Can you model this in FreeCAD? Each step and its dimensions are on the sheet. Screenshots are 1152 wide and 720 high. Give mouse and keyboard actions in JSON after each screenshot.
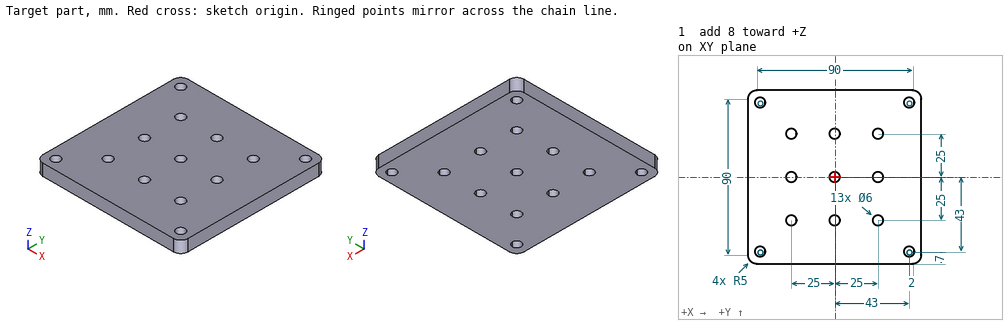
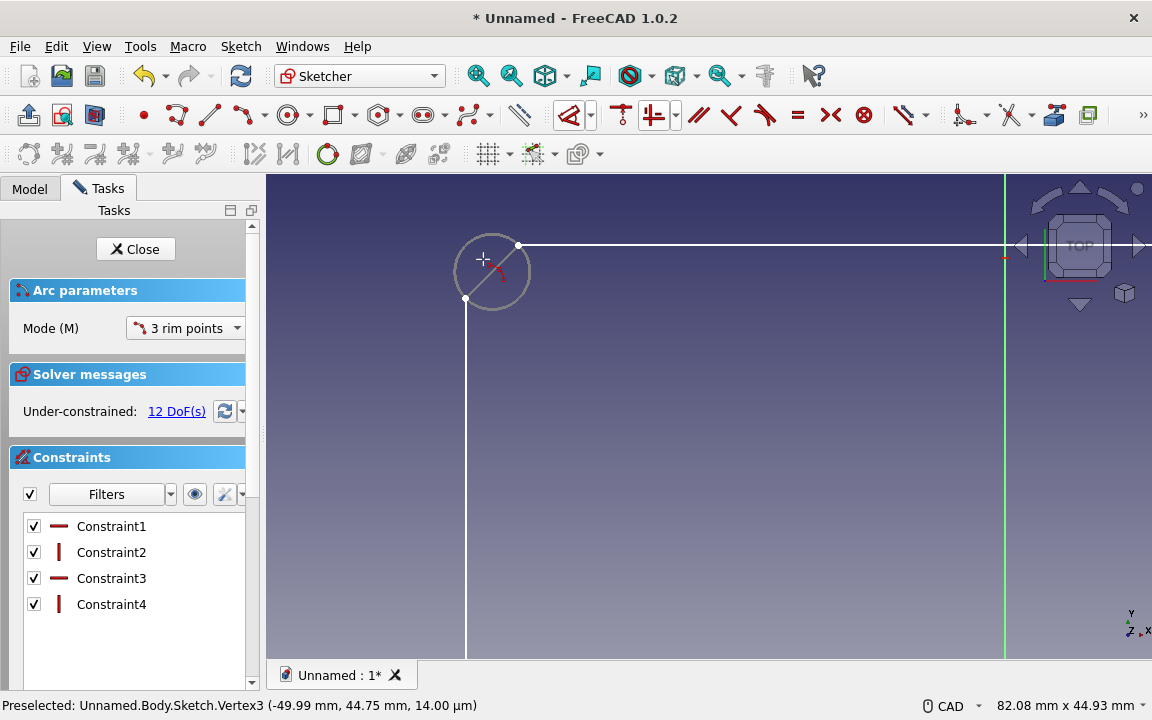
{"action": "left_click", "coordinate": [481, 257]}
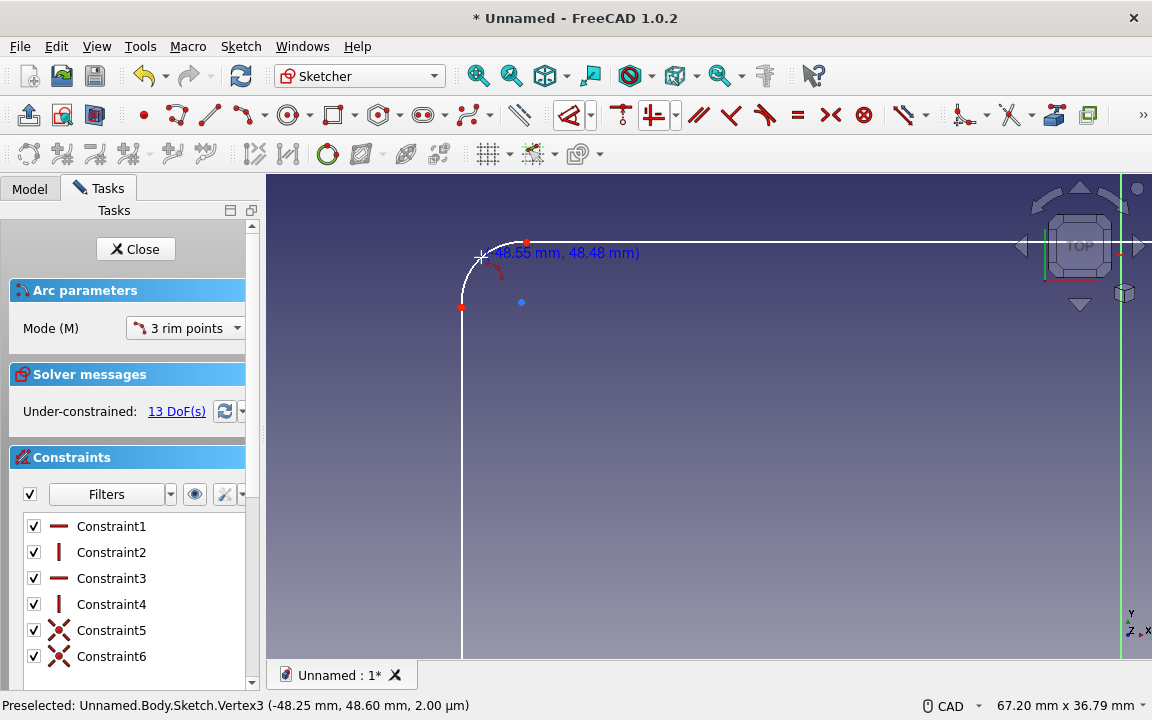
{"action": "scroll", "coordinate": [483, 259], "scroll_direction": "down", "scroll_amount": 7}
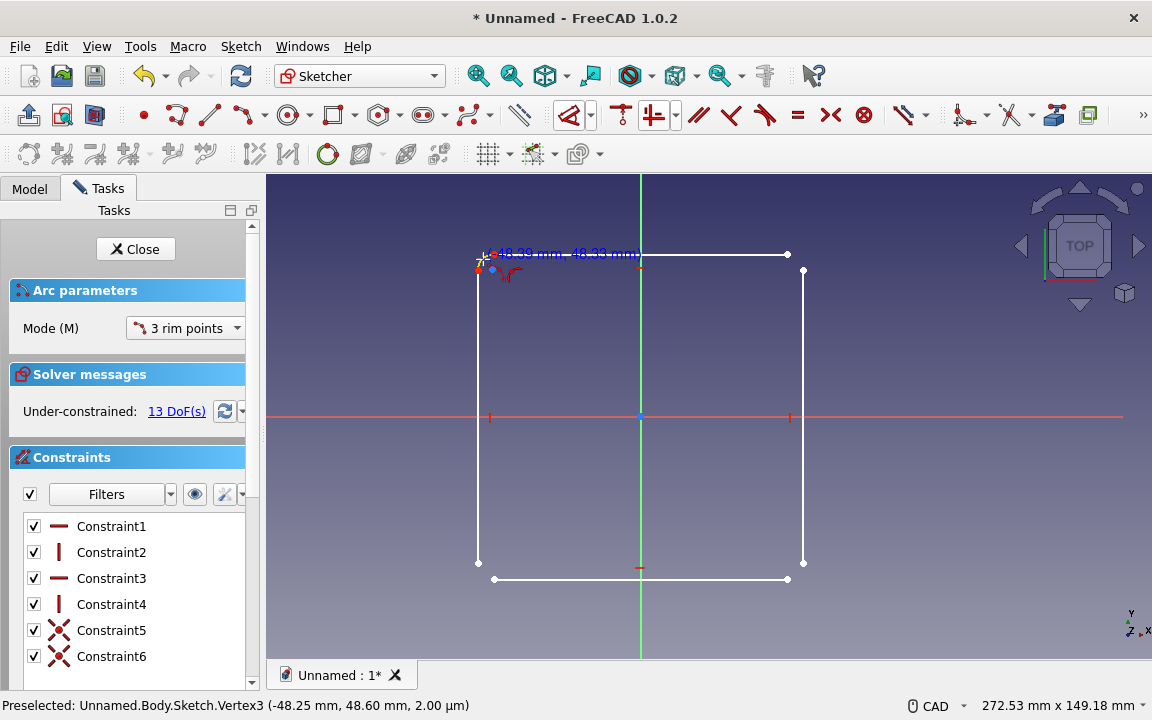
{"action": "left_click", "coordinate": [478, 564]}
{"action": "left_click", "coordinate": [494, 580]}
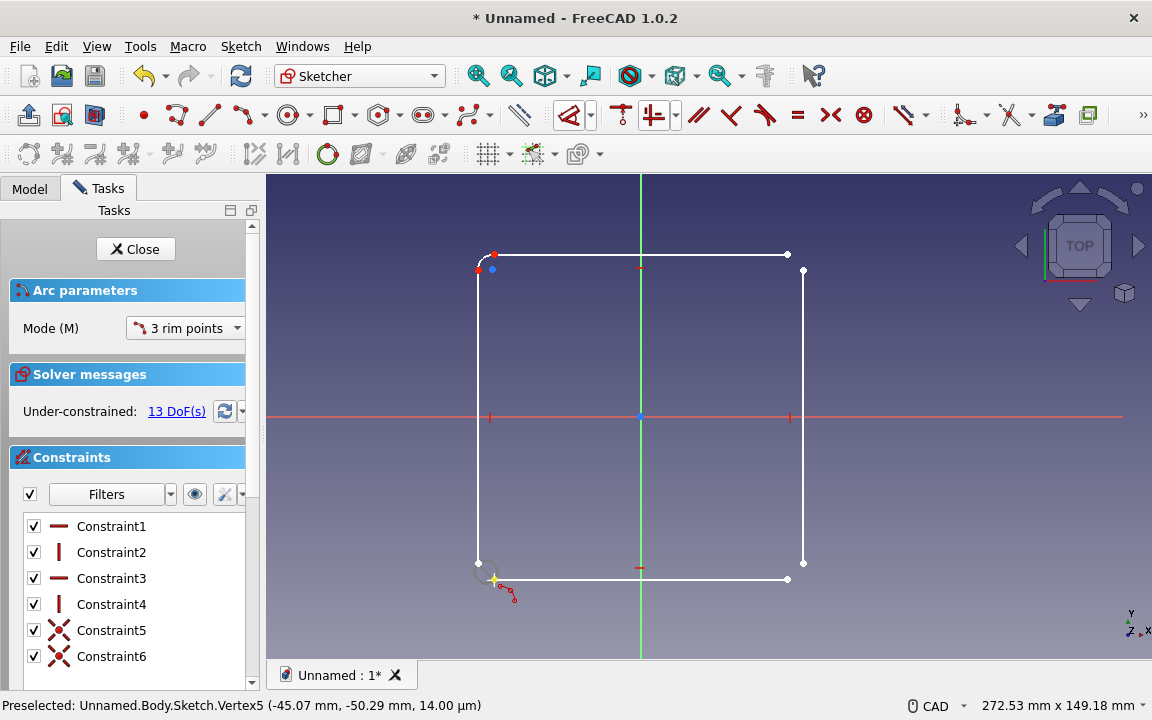
{"action": "scroll", "coordinate": [483, 574], "scroll_direction": "up", "scroll_amount": 7}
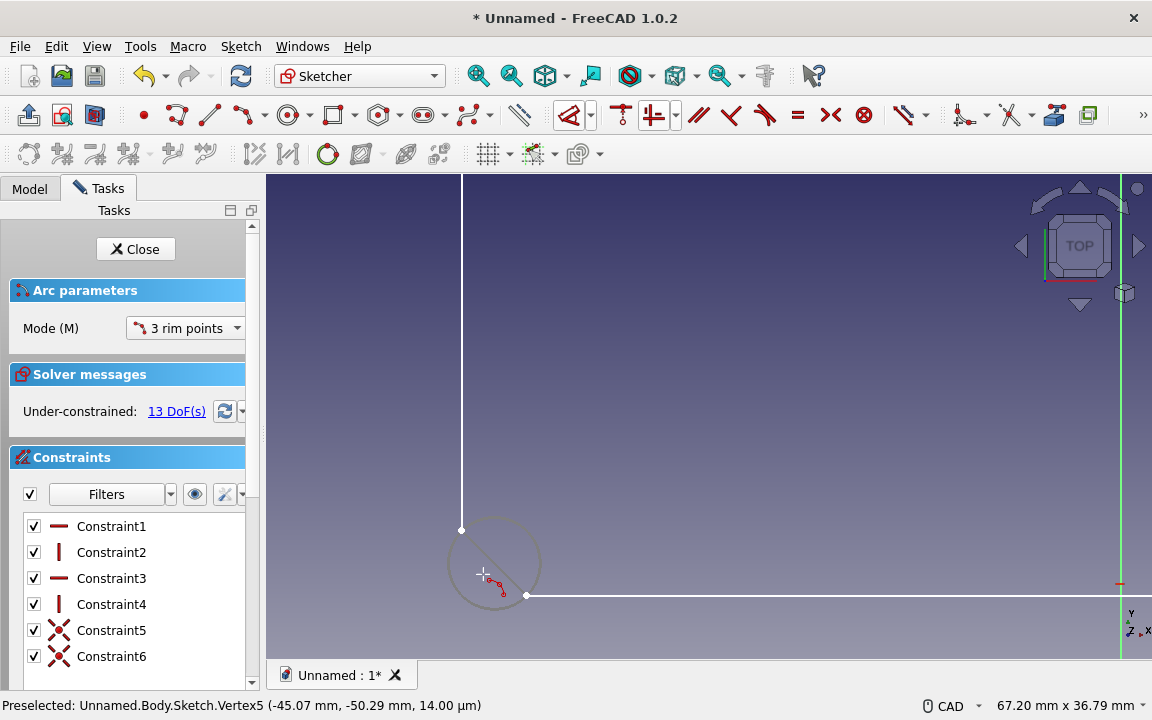
{"action": "left_click", "coordinate": [481, 573]}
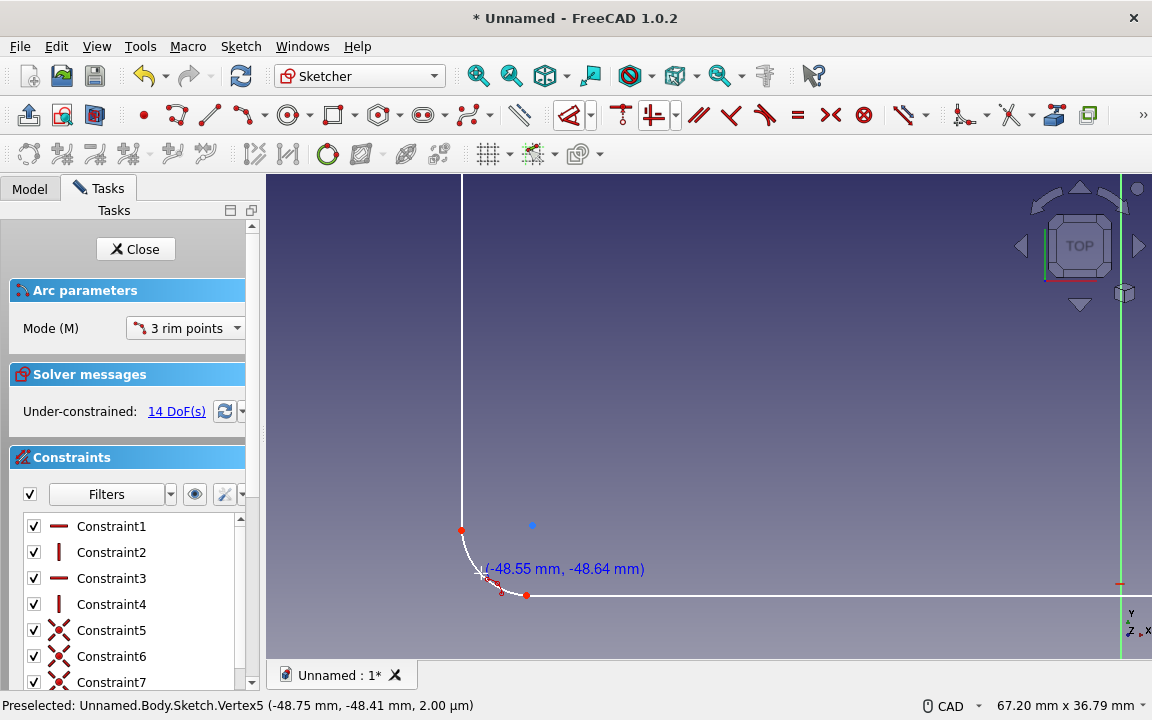
{"action": "scroll", "coordinate": [483, 575], "scroll_direction": "down", "scroll_amount": 7}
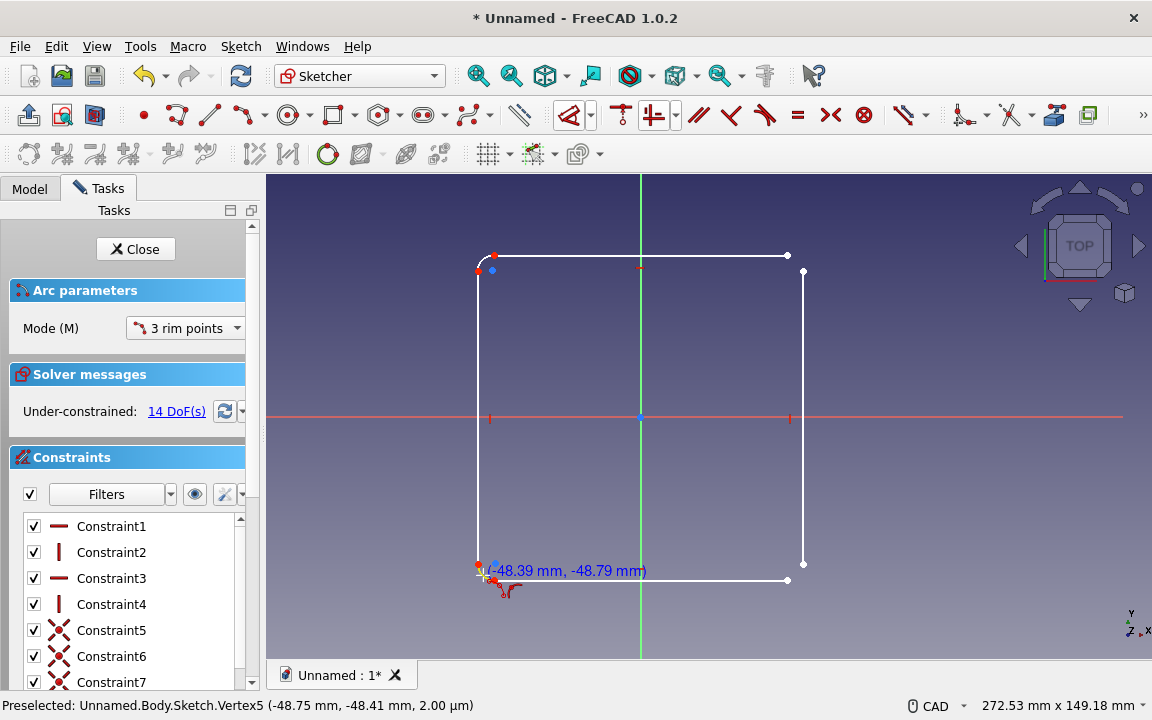
{"action": "left_click", "coordinate": [787, 581]}
{"action": "left_click", "coordinate": [803, 565]}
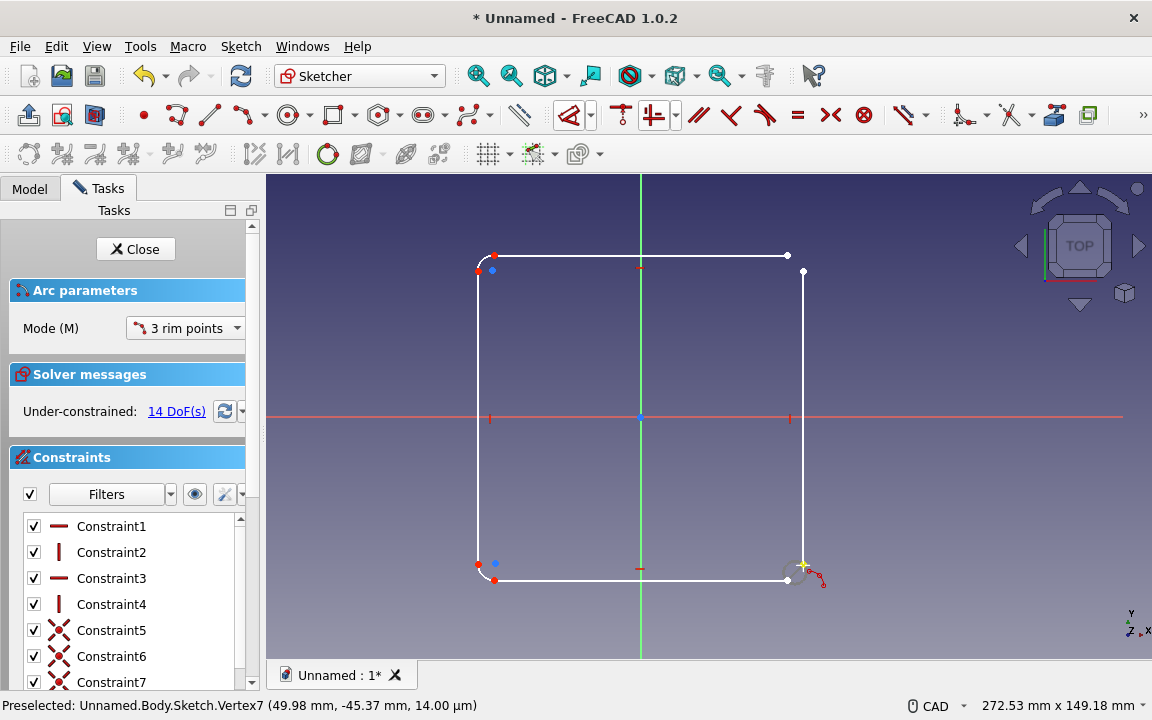
{"action": "scroll", "coordinate": [798, 575], "scroll_direction": "up", "scroll_amount": 7}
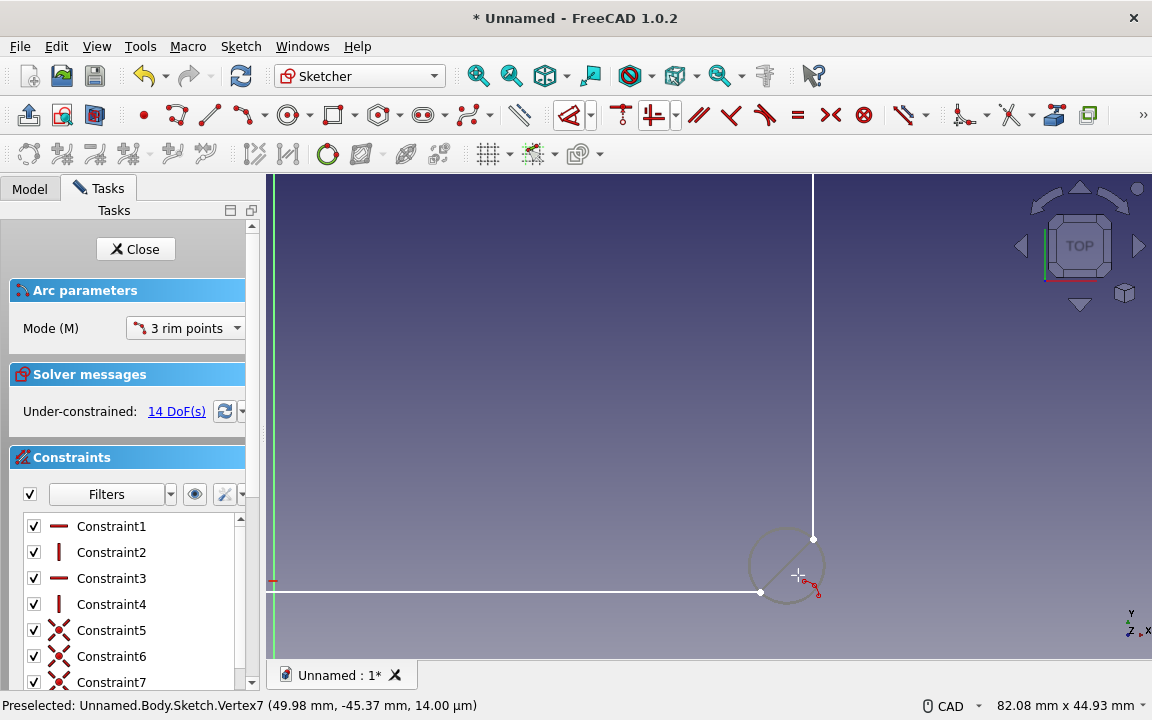
{"action": "left_click", "coordinate": [797, 573]}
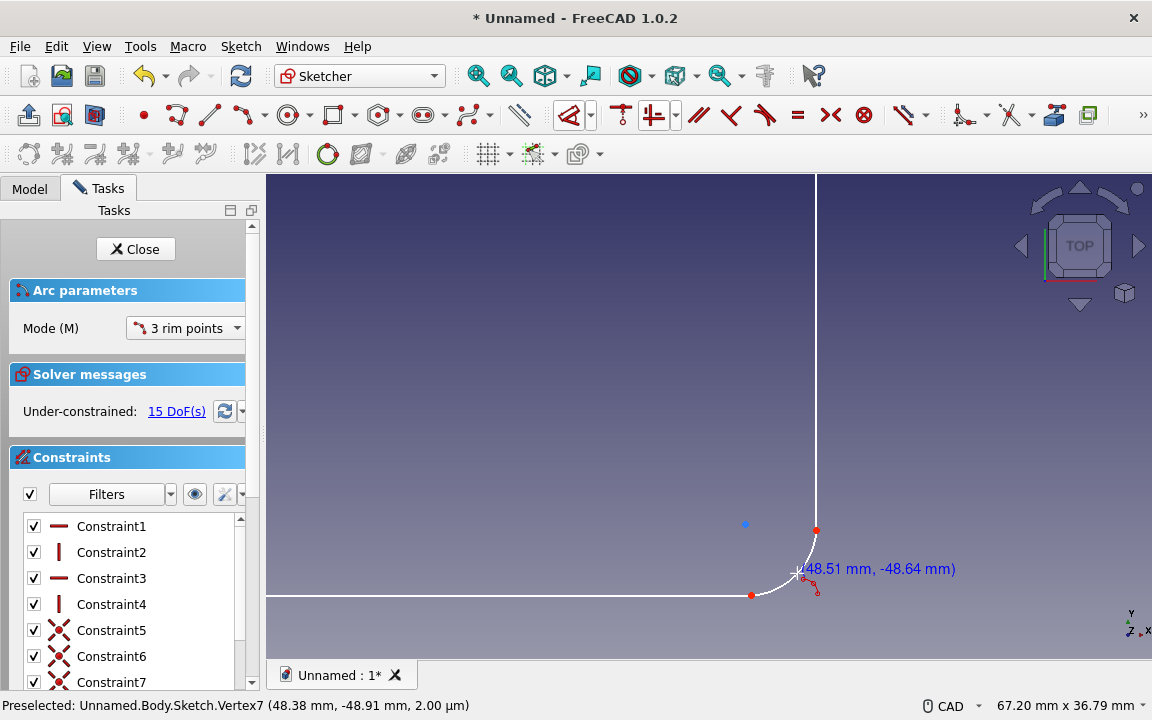
{"action": "scroll", "coordinate": [799, 575], "scroll_direction": "down", "scroll_amount": 7}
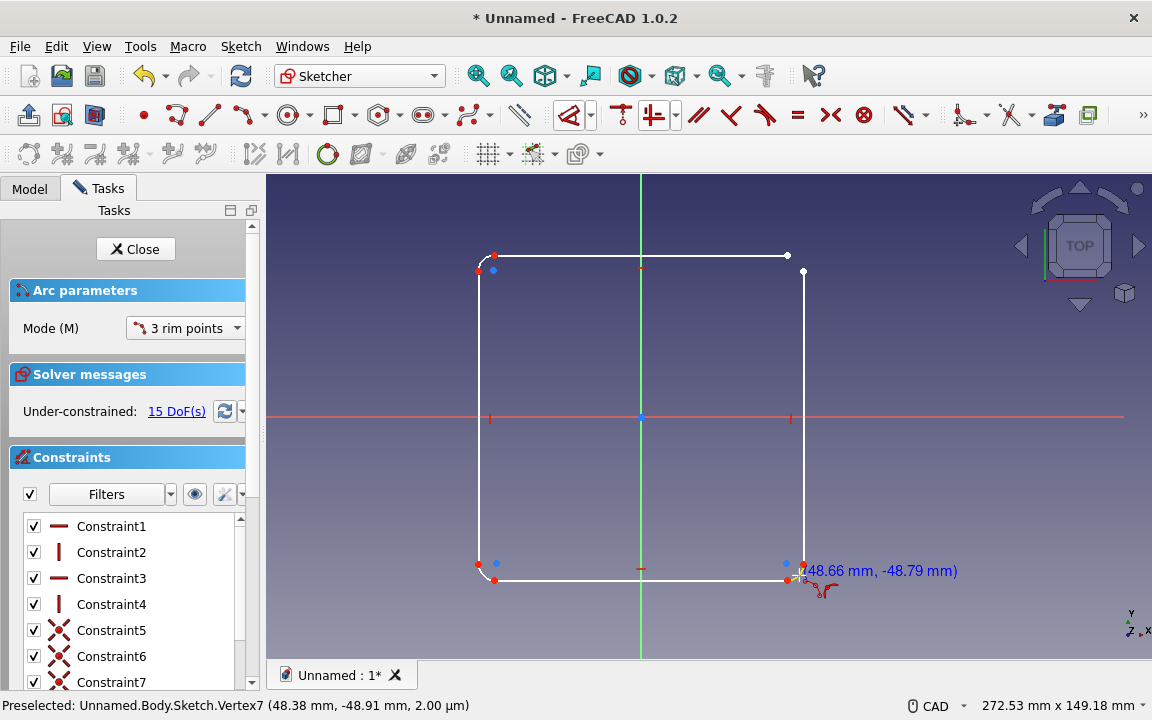
{"action": "left_click", "coordinate": [804, 272]}
{"action": "left_click", "coordinate": [788, 256]}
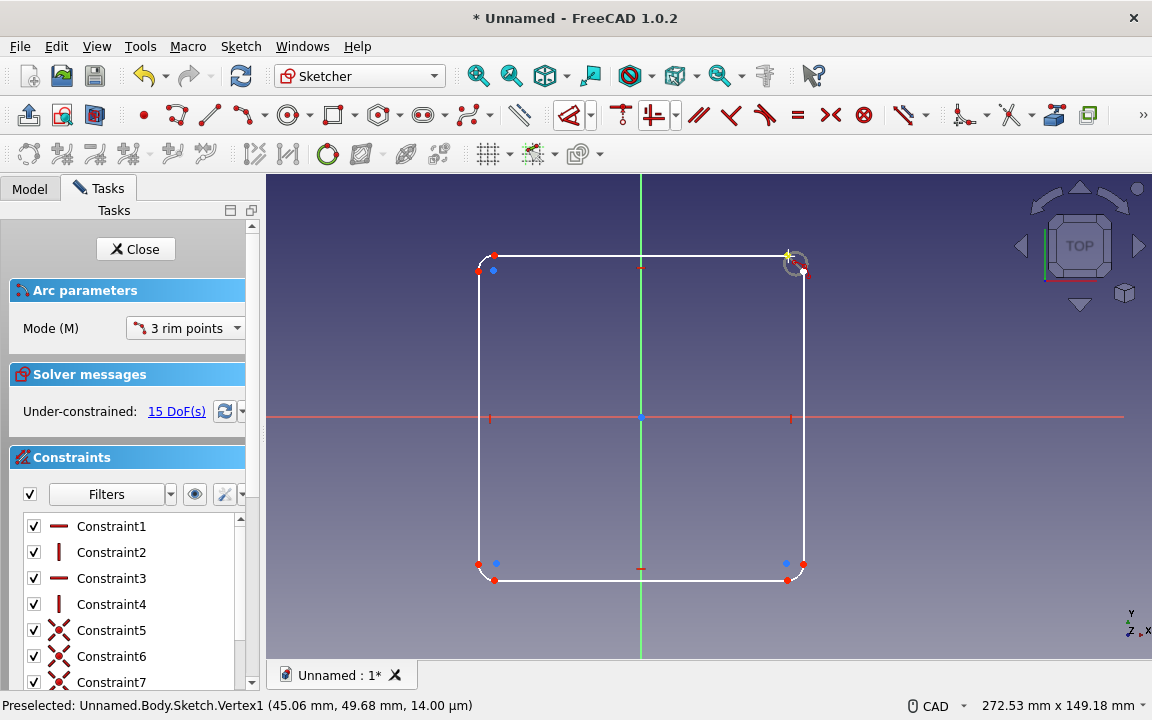
{"action": "scroll", "coordinate": [799, 259], "scroll_direction": "up", "scroll_amount": 7}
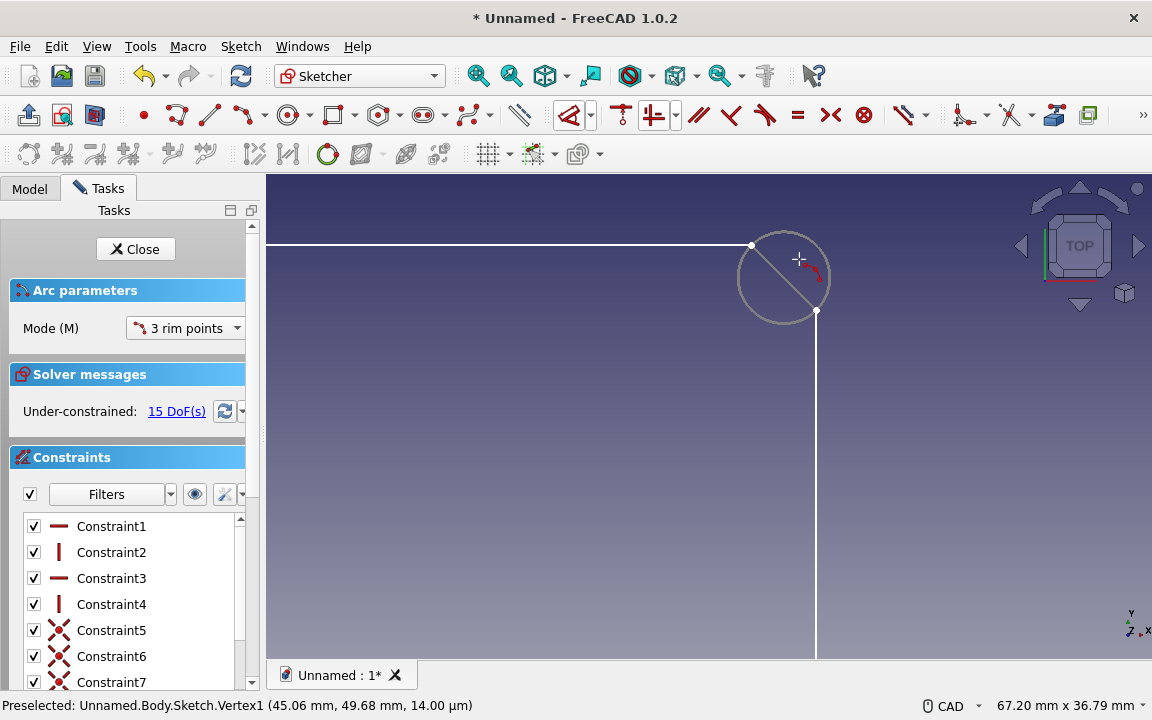
{"action": "left_click", "coordinate": [797, 260]}